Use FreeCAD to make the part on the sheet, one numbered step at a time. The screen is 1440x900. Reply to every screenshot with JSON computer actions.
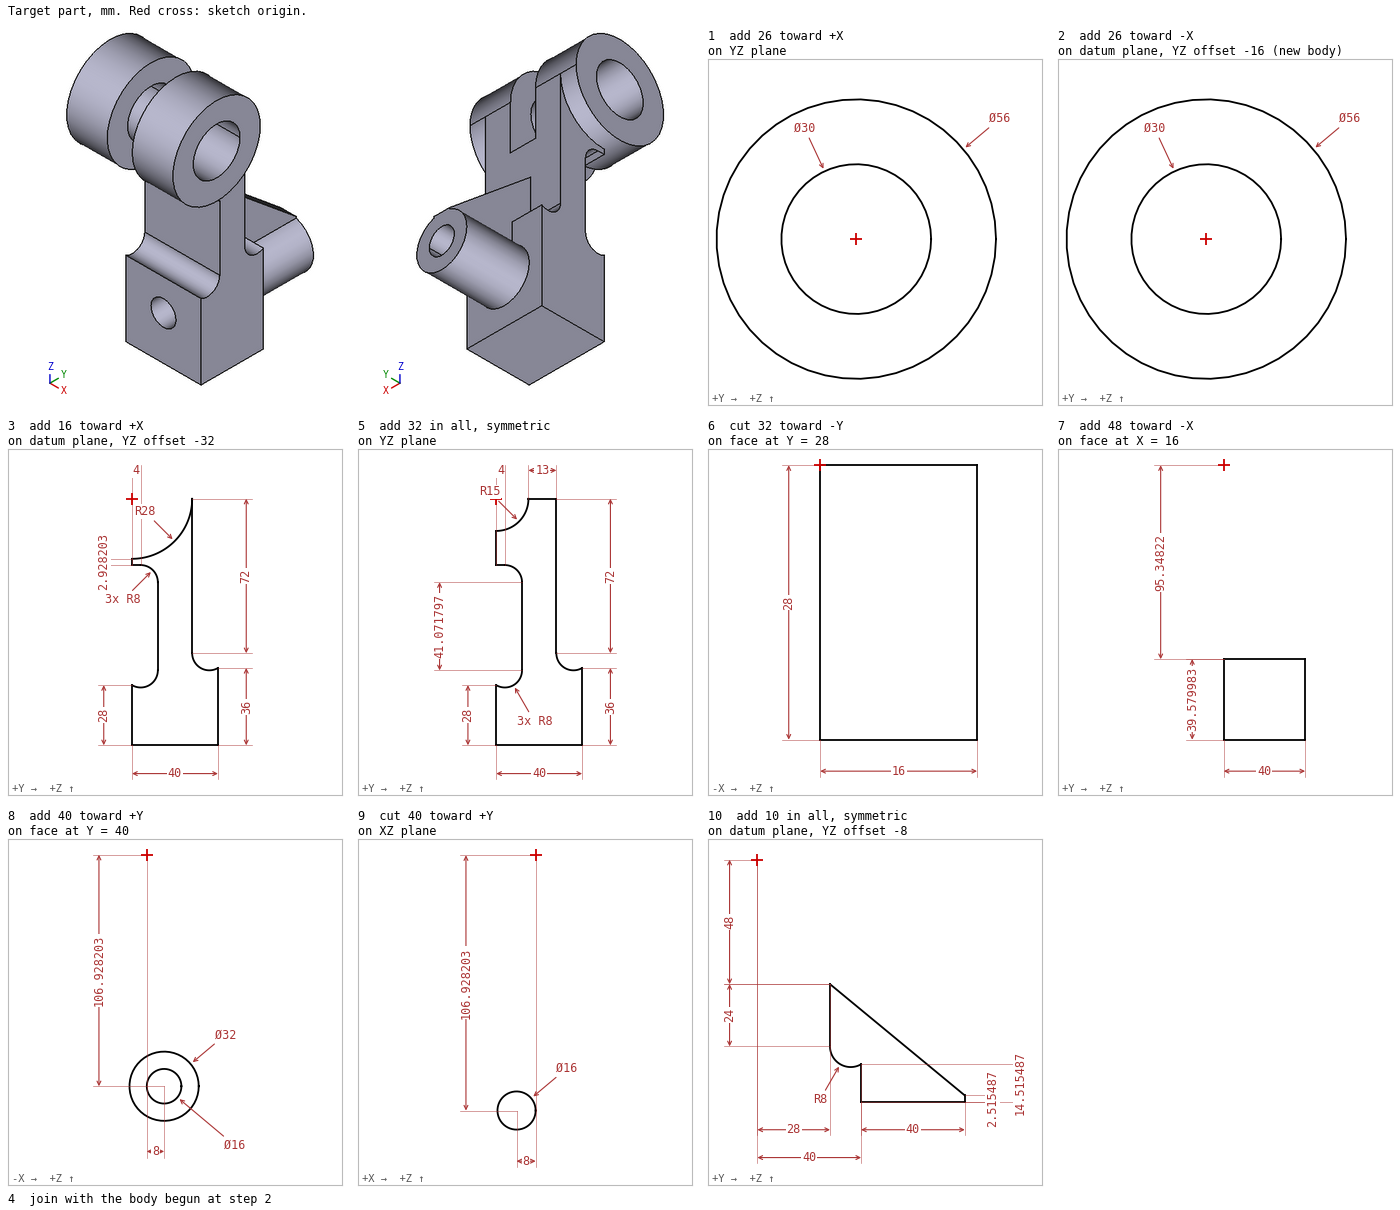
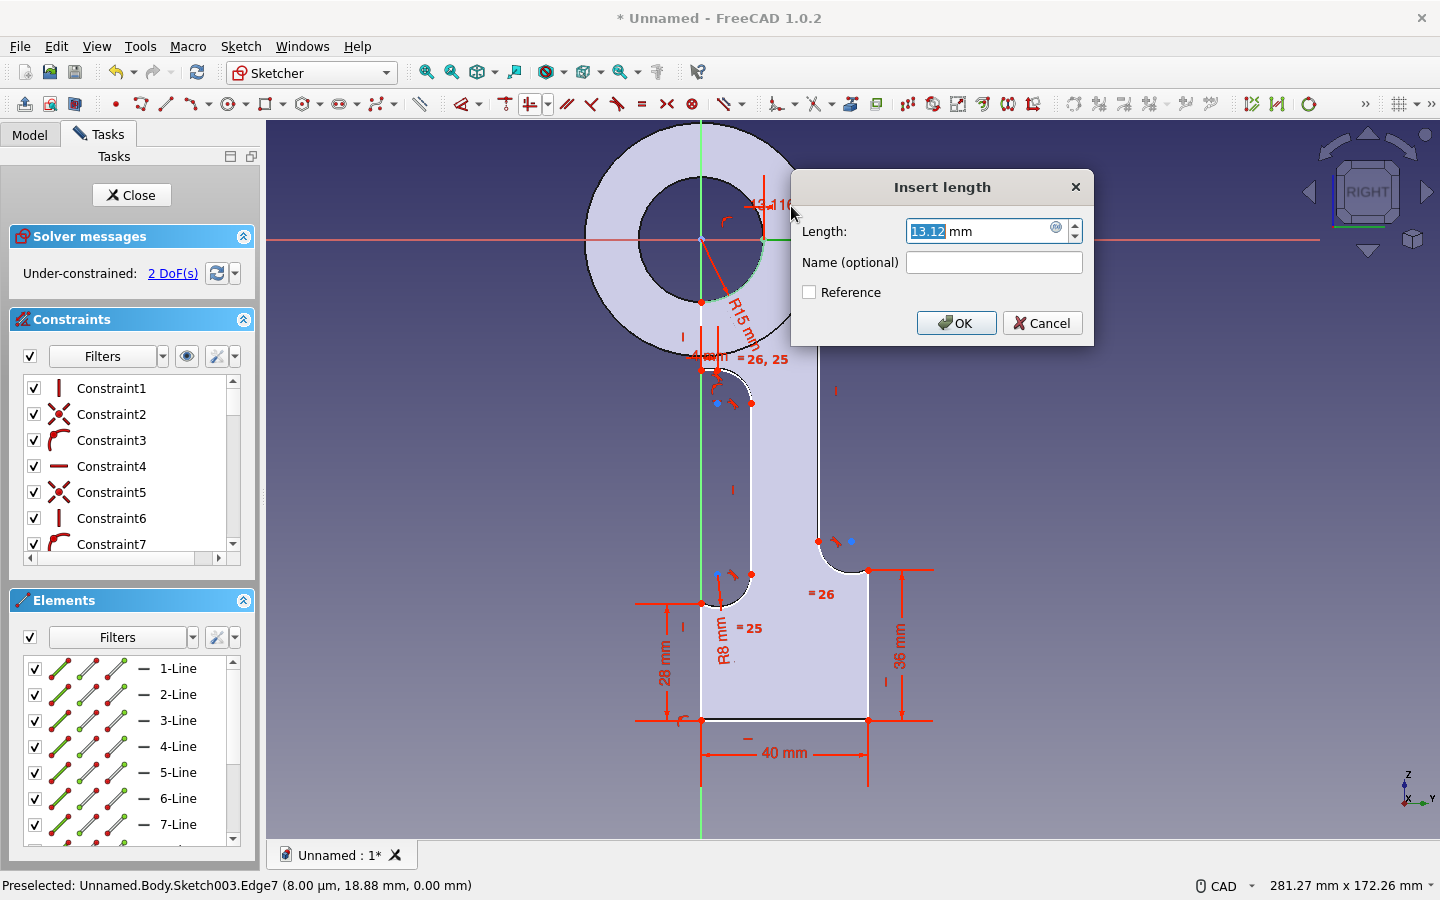
{"action": "type", "text": "13"}
{"action": "key", "text": "Return"}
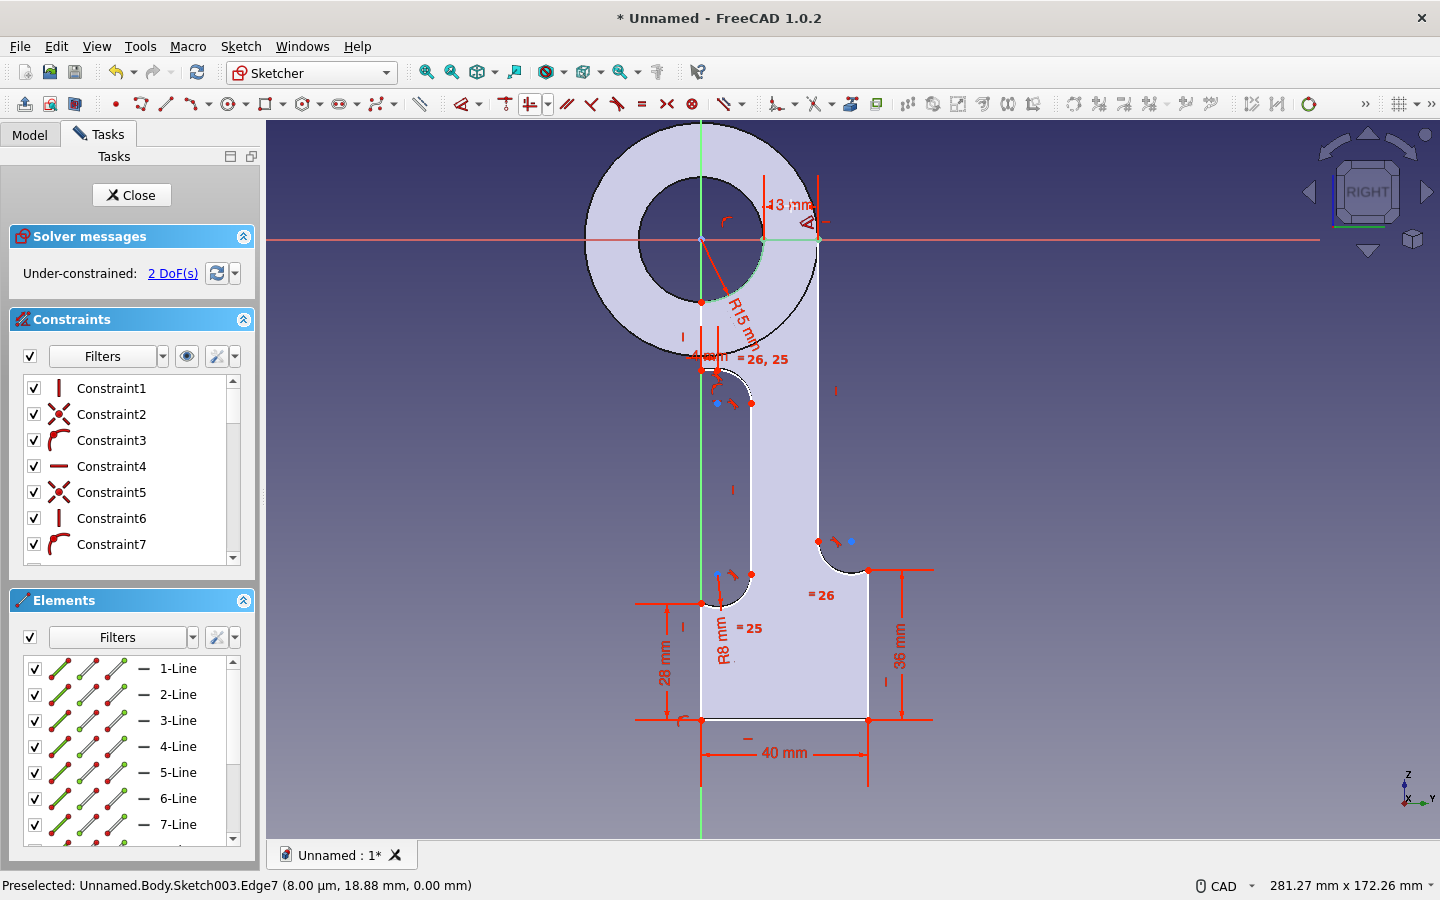
{"action": "left_click", "coordinate": [818, 330]}
{"action": "left_click", "coordinate": [852, 390]}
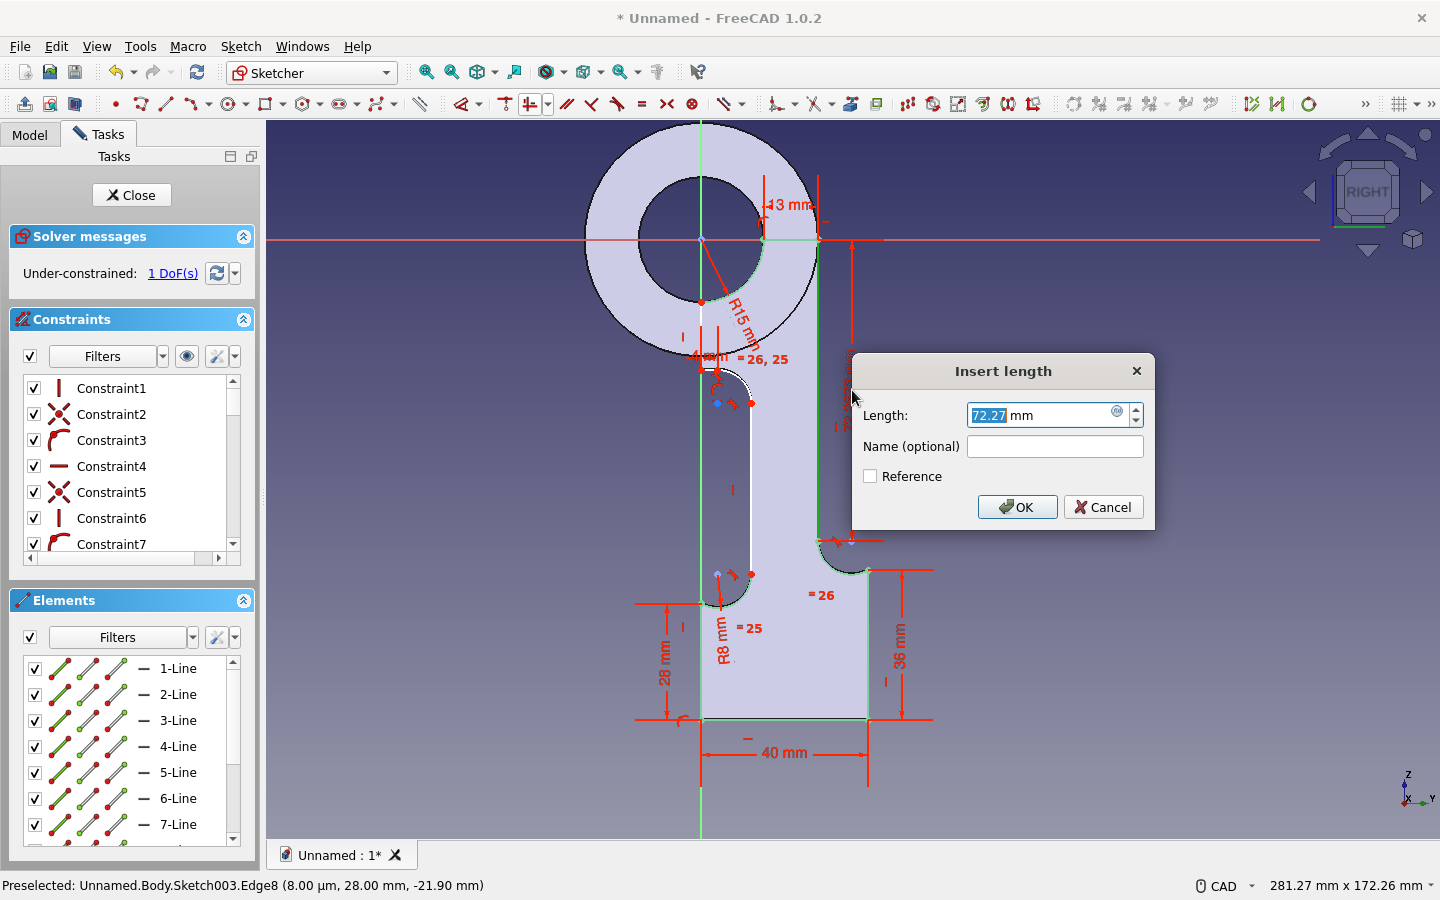
{"action": "type", "text": "72"}
{"action": "key", "text": "Return"}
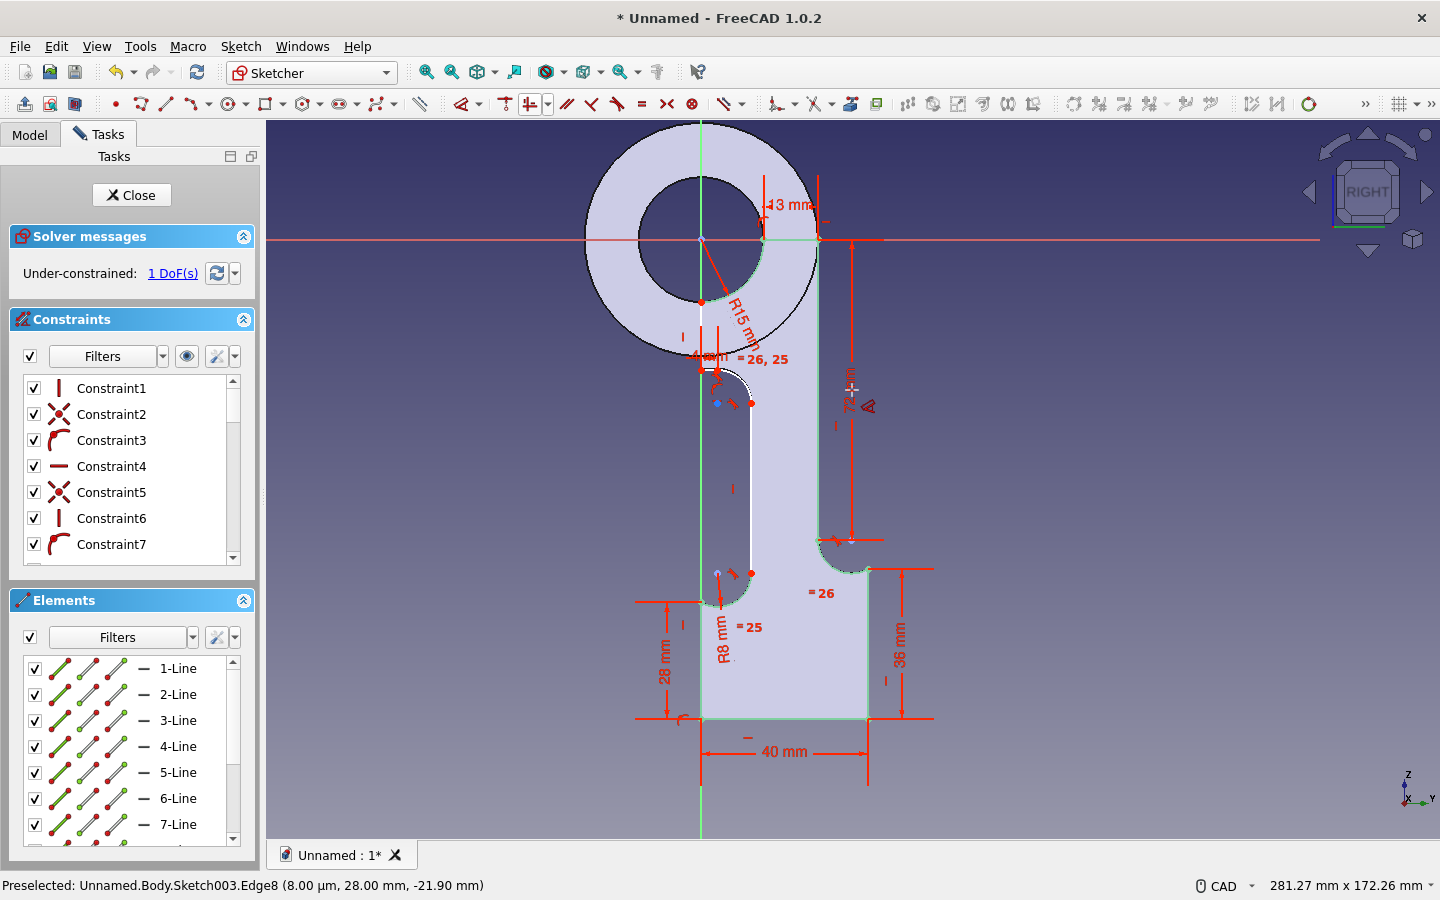
{"action": "left_click", "coordinate": [751, 523]}
{"action": "left_click", "coordinate": [717, 489]}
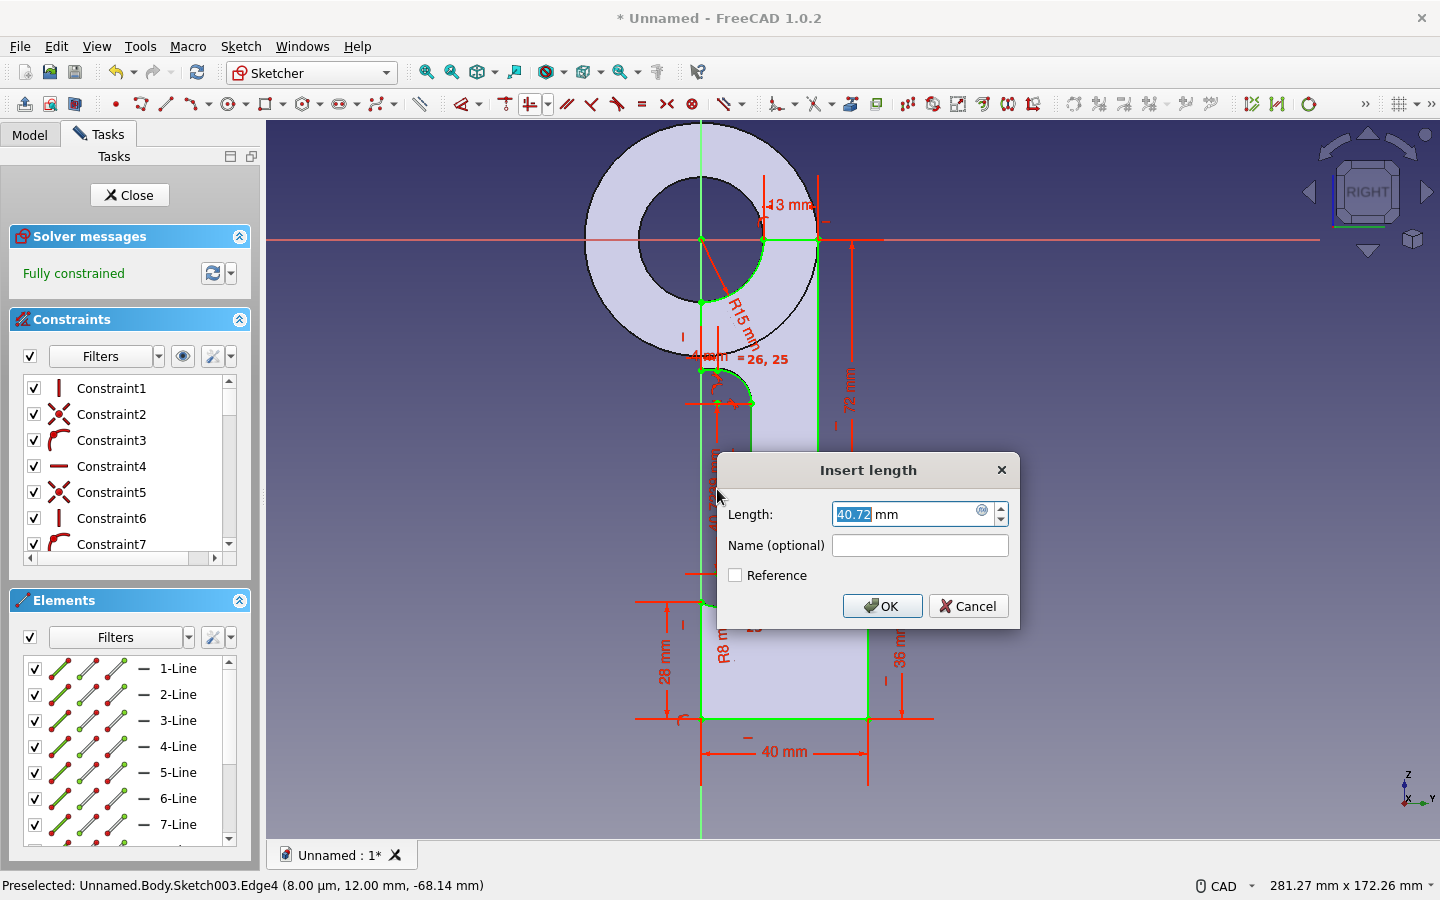
{"action": "type", "text": "41.071797"}
{"action": "key", "text": "Return"}
{"action": "key", "text": "Escape"}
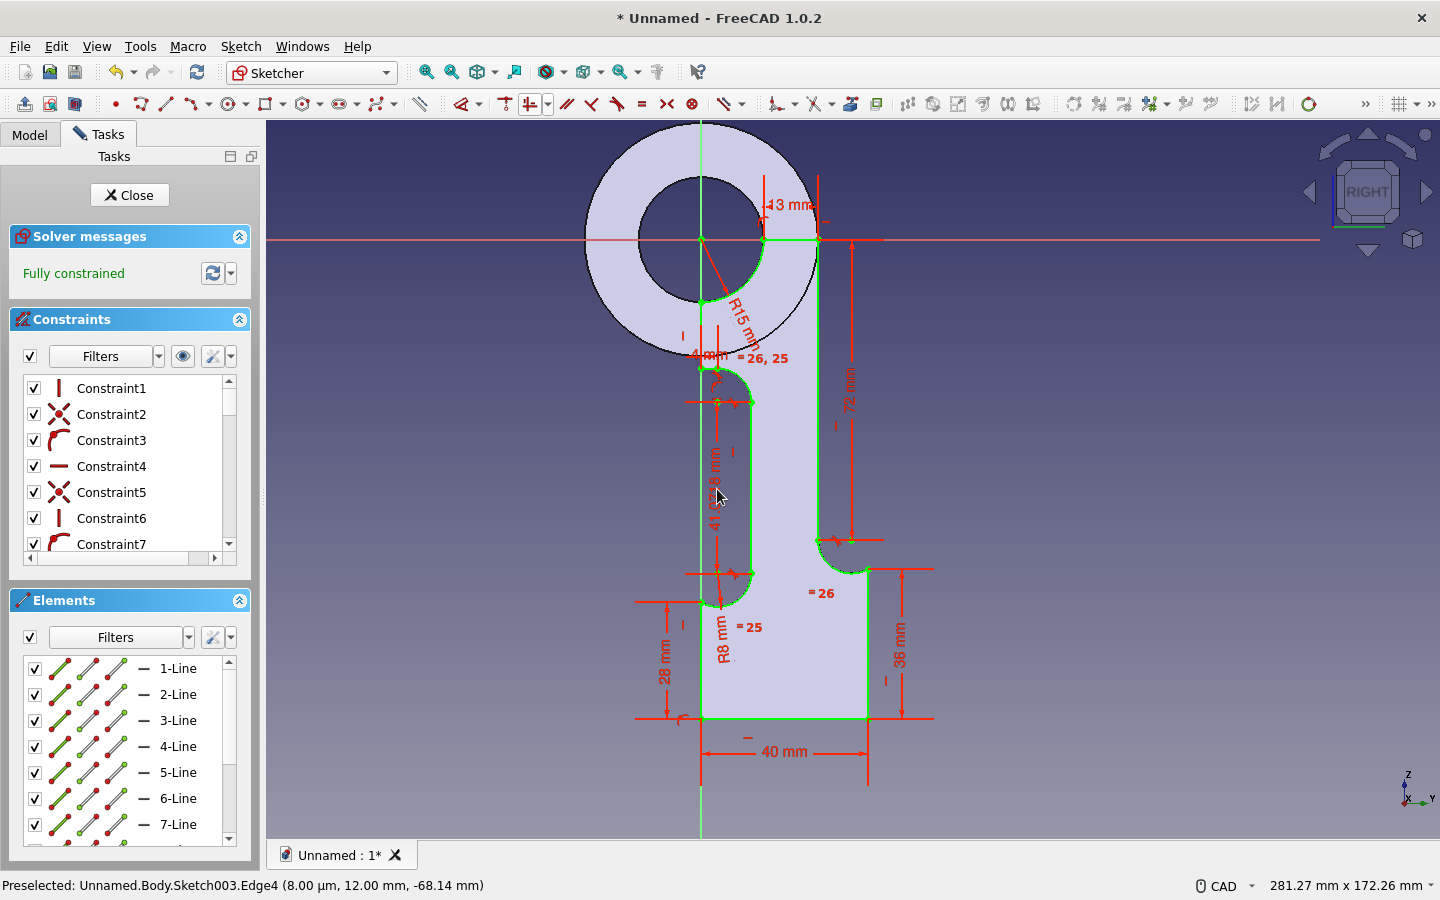
{"action": "left_click", "coordinate": [130, 195]}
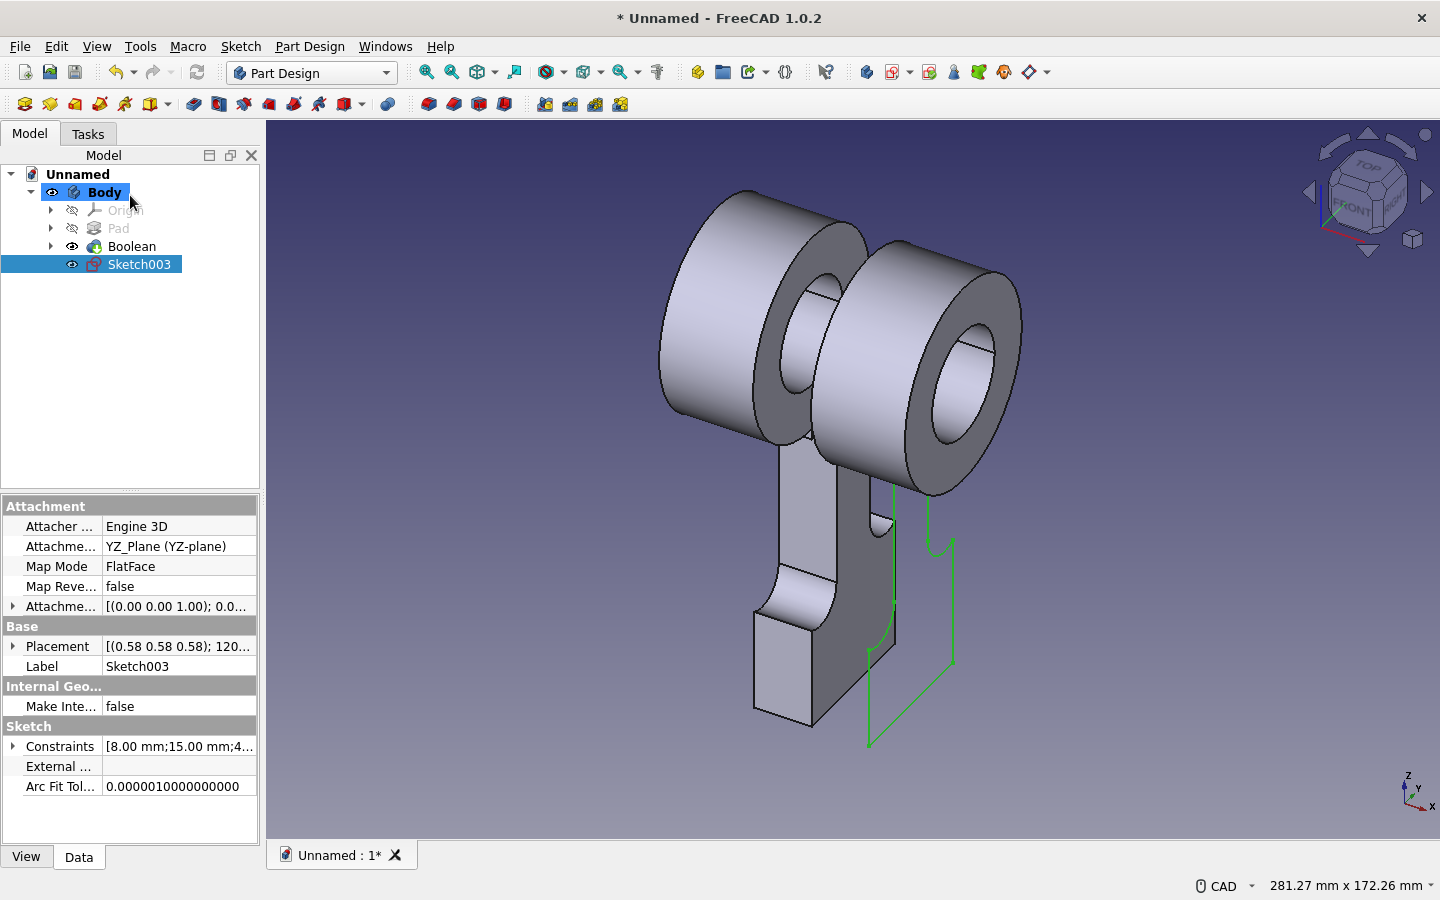
{"action": "left_click", "coordinate": [25, 104]}